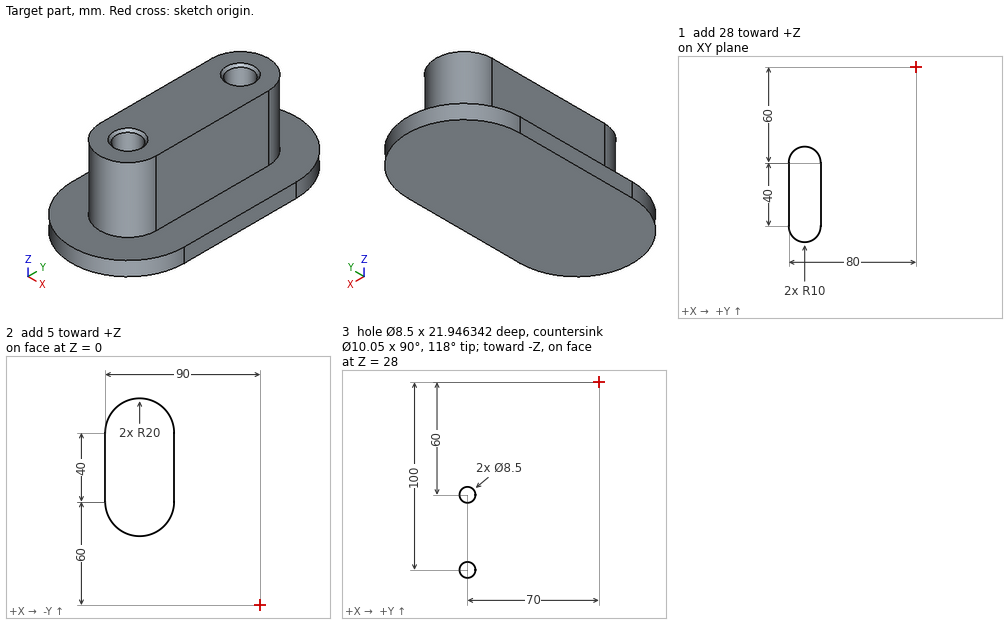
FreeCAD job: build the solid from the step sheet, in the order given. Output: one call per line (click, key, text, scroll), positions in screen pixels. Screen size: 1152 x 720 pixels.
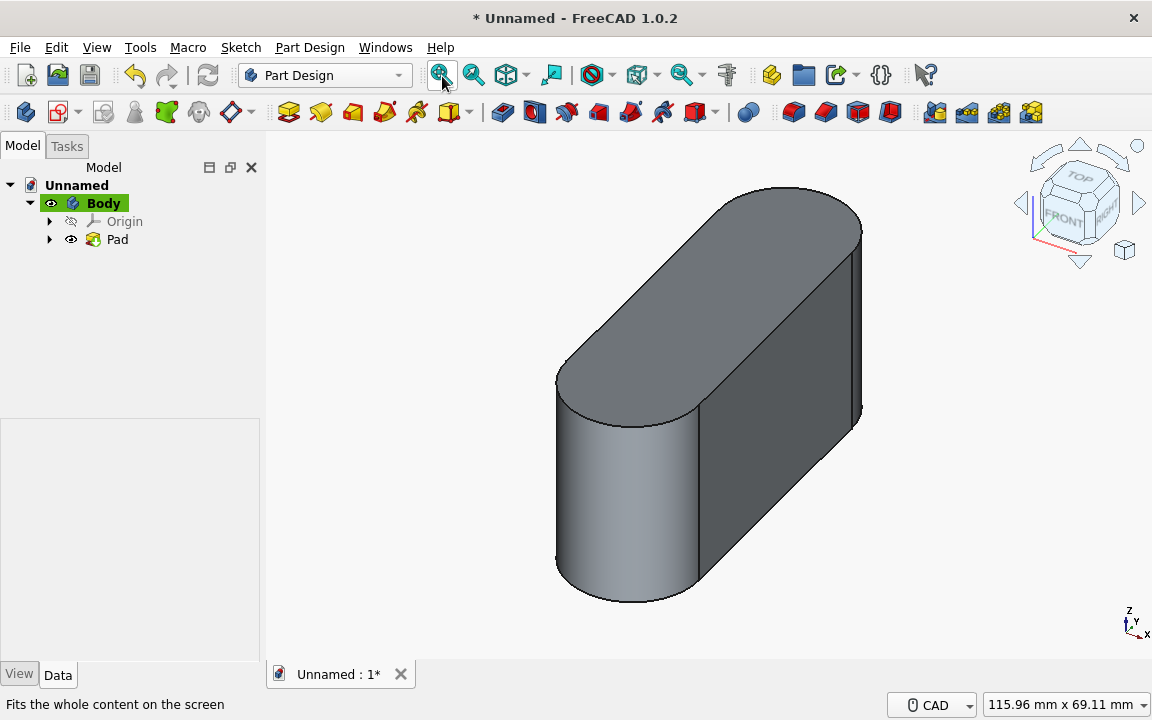
key(5)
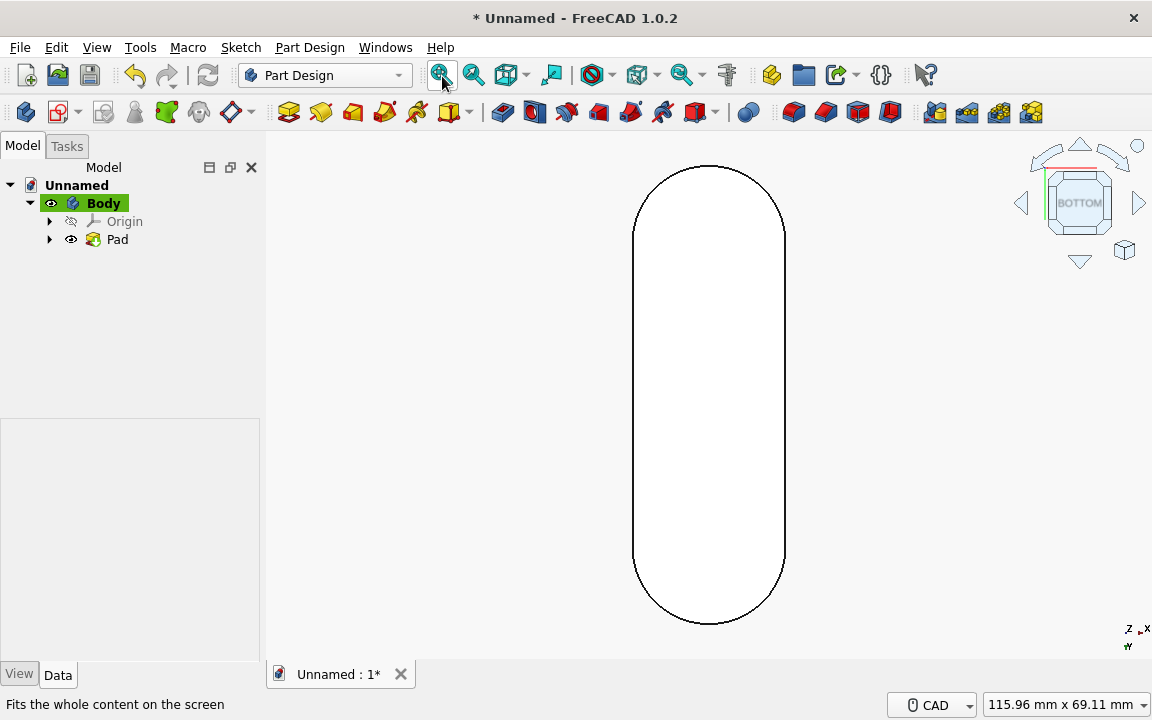
click(709, 525)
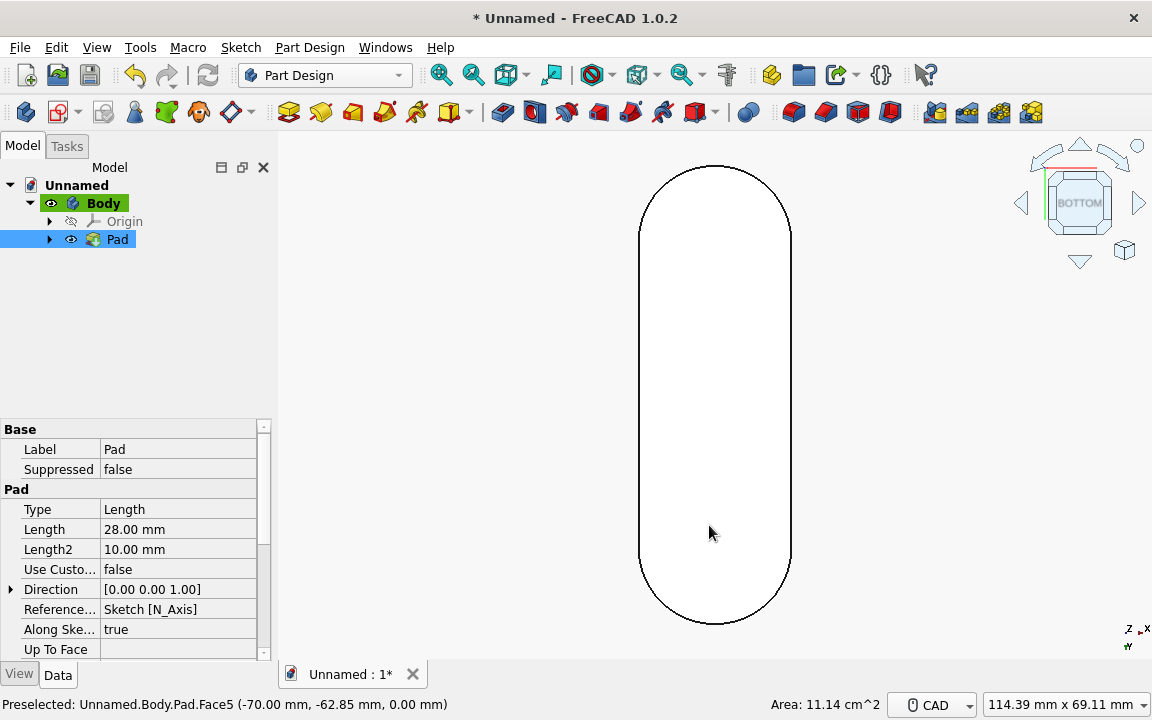
click(58, 112)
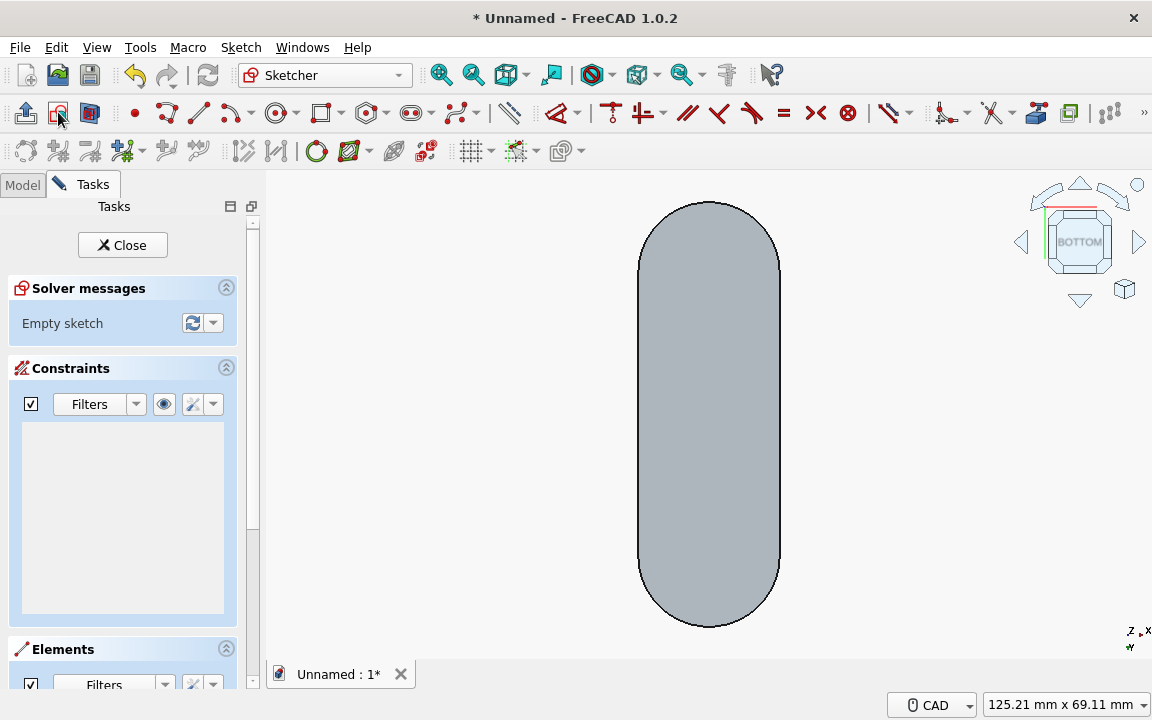
scroll(498, 332, down, 5)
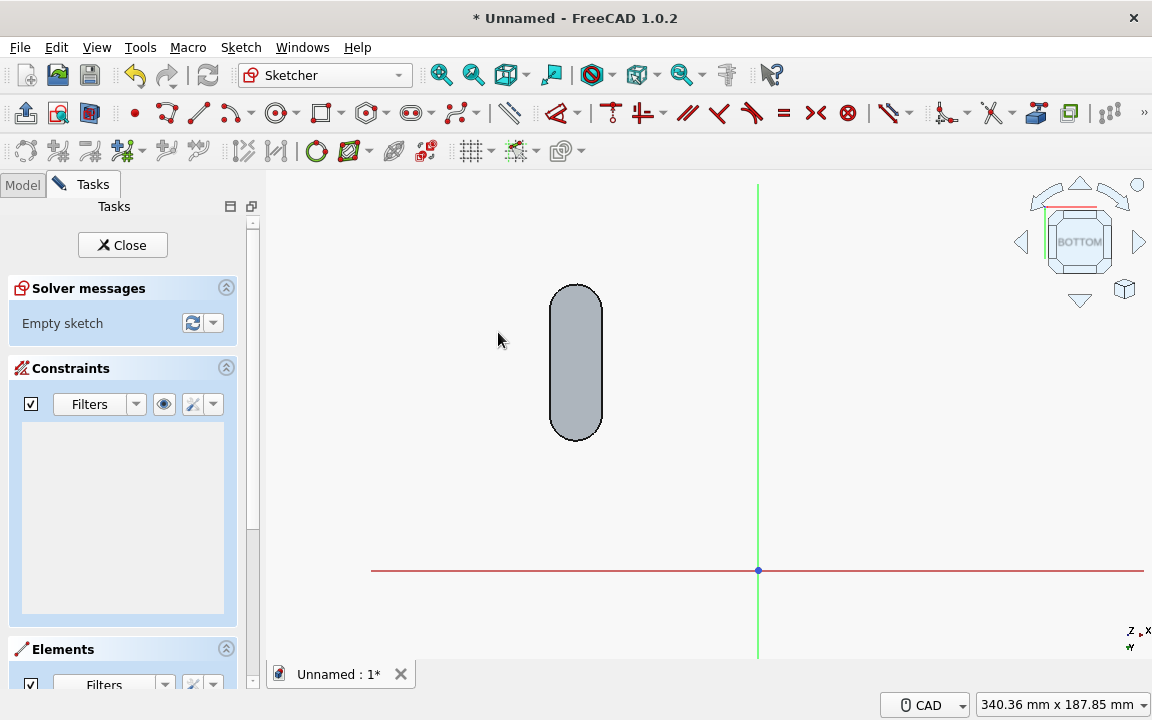
click(412, 114)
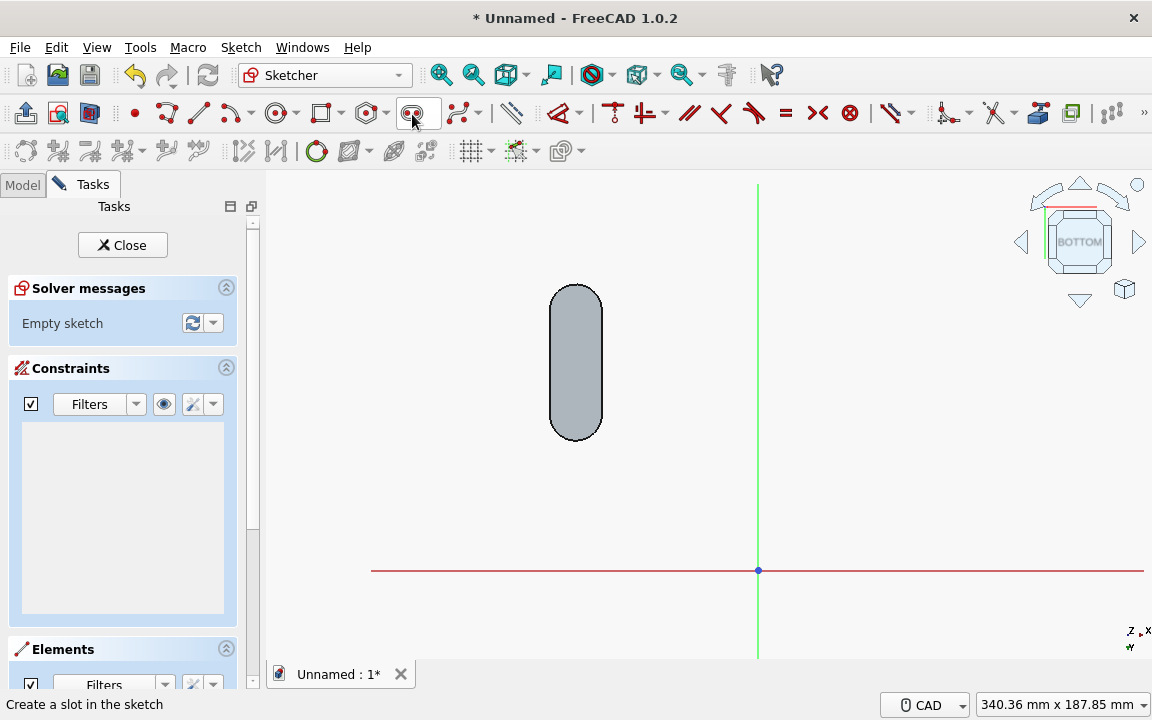
click(576, 415)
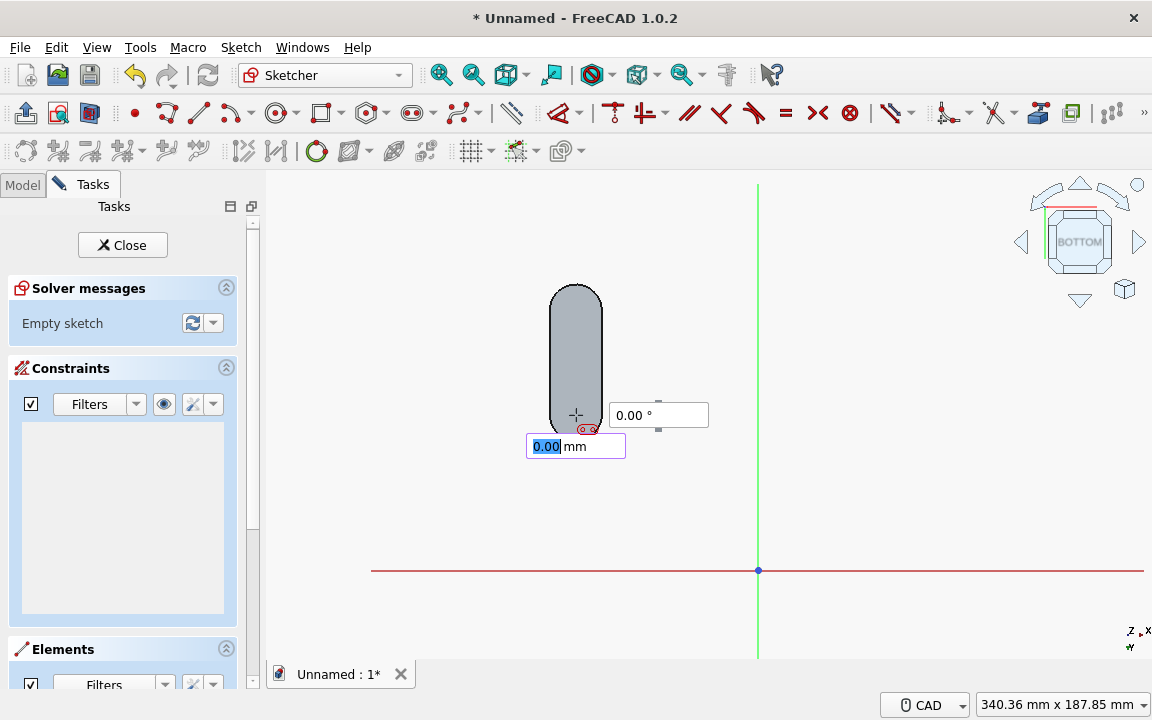
click(576, 310)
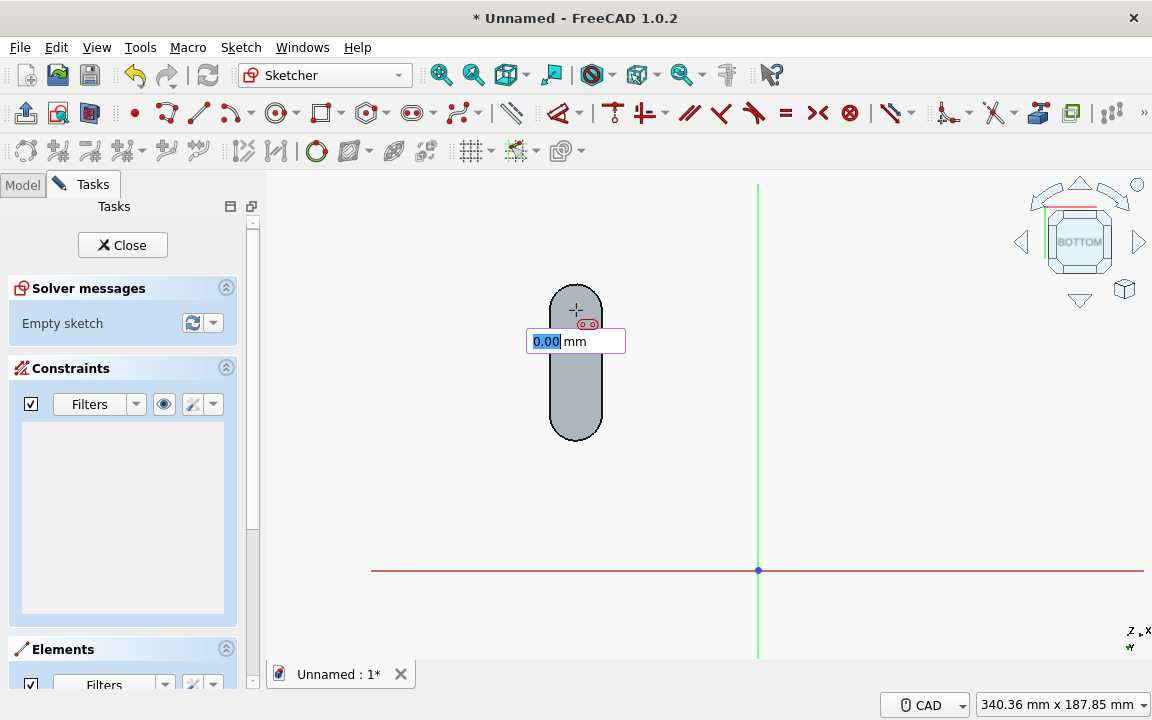
click(524, 363)
key(Escape)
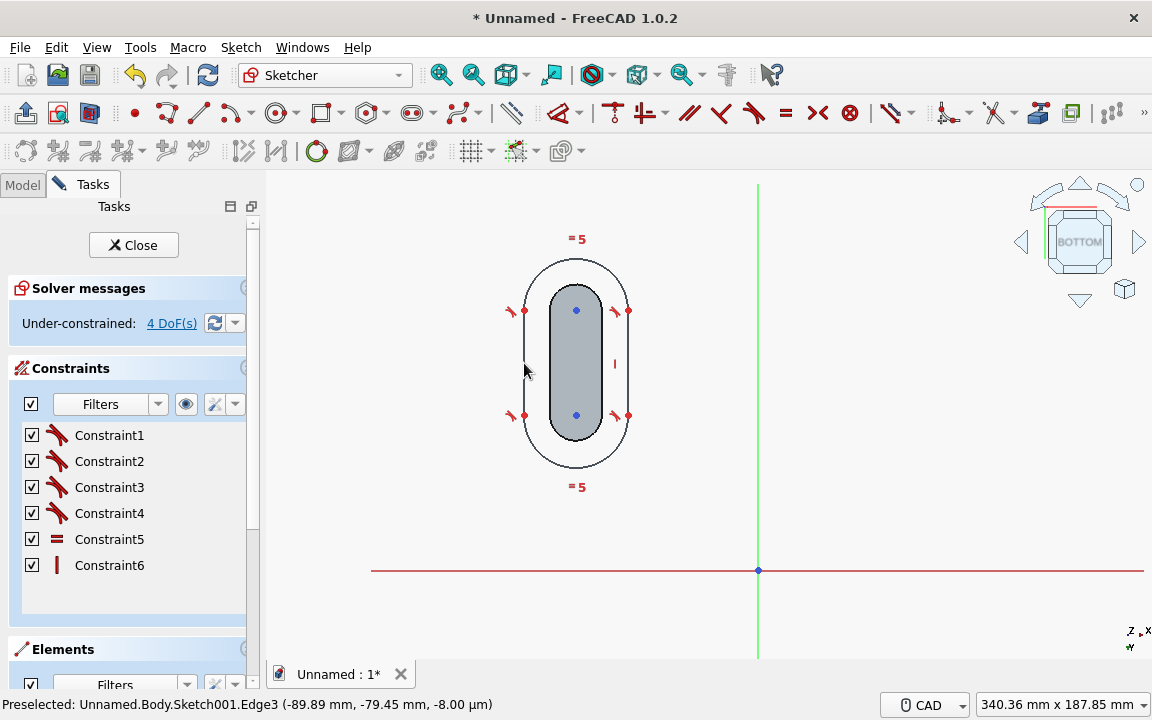
click(558, 114)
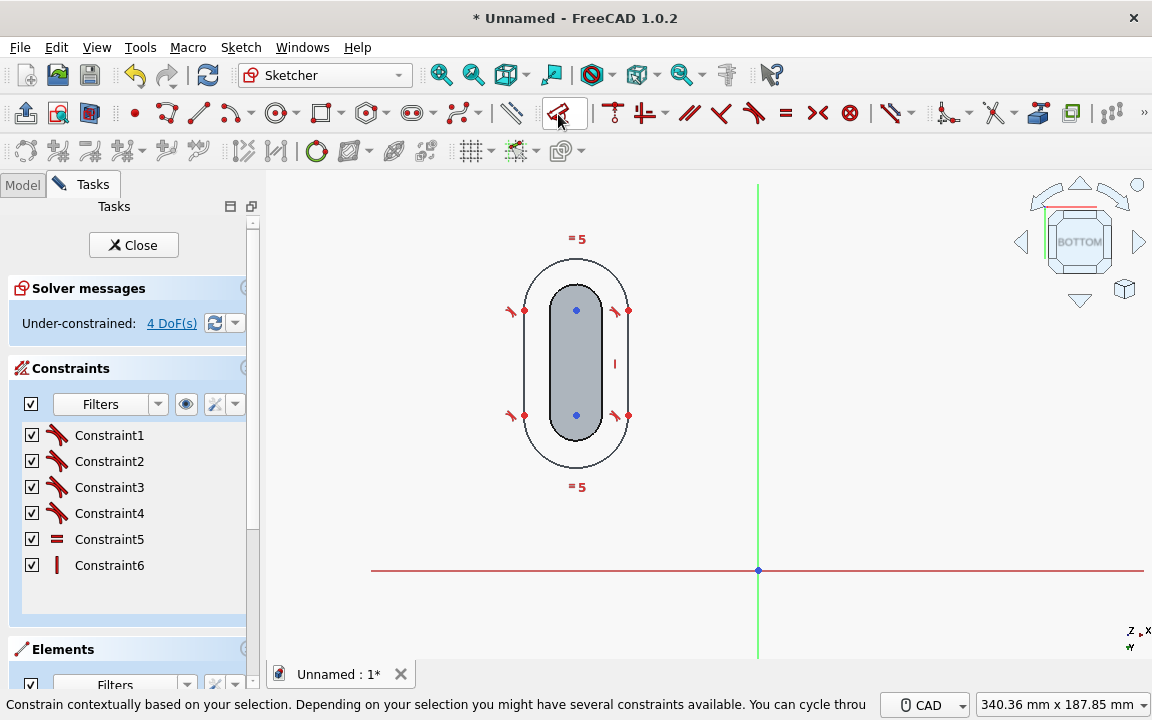
click(545, 458)
click(526, 484)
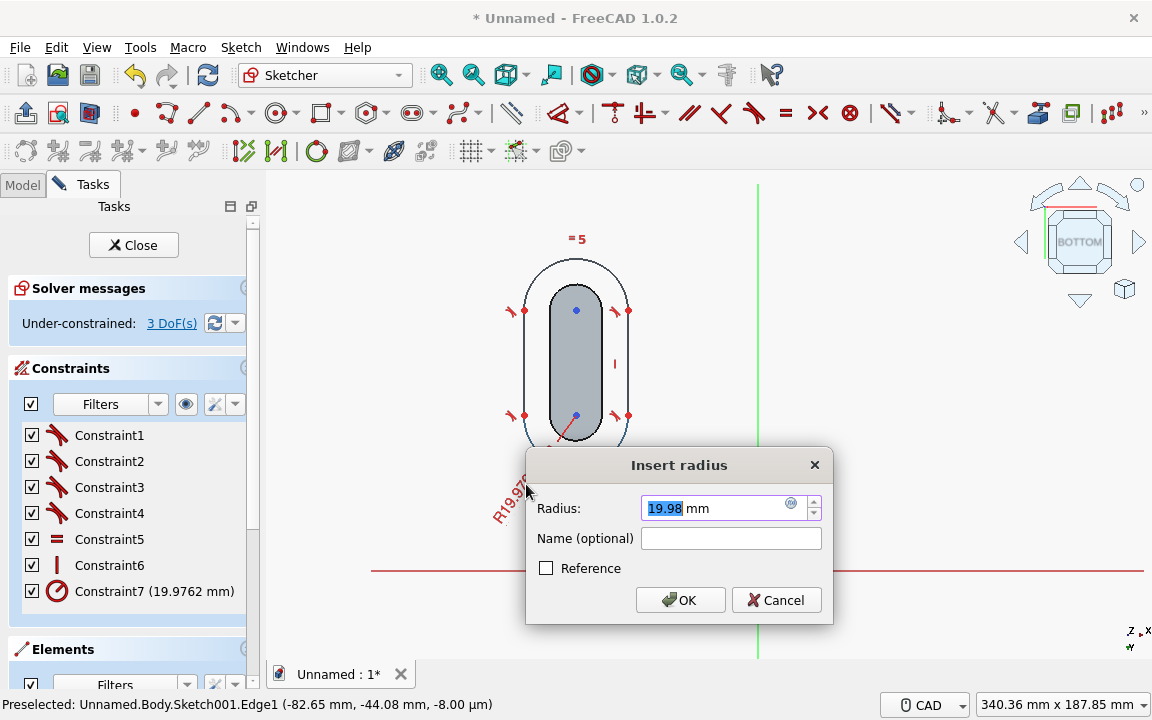
text(20)
key(Return)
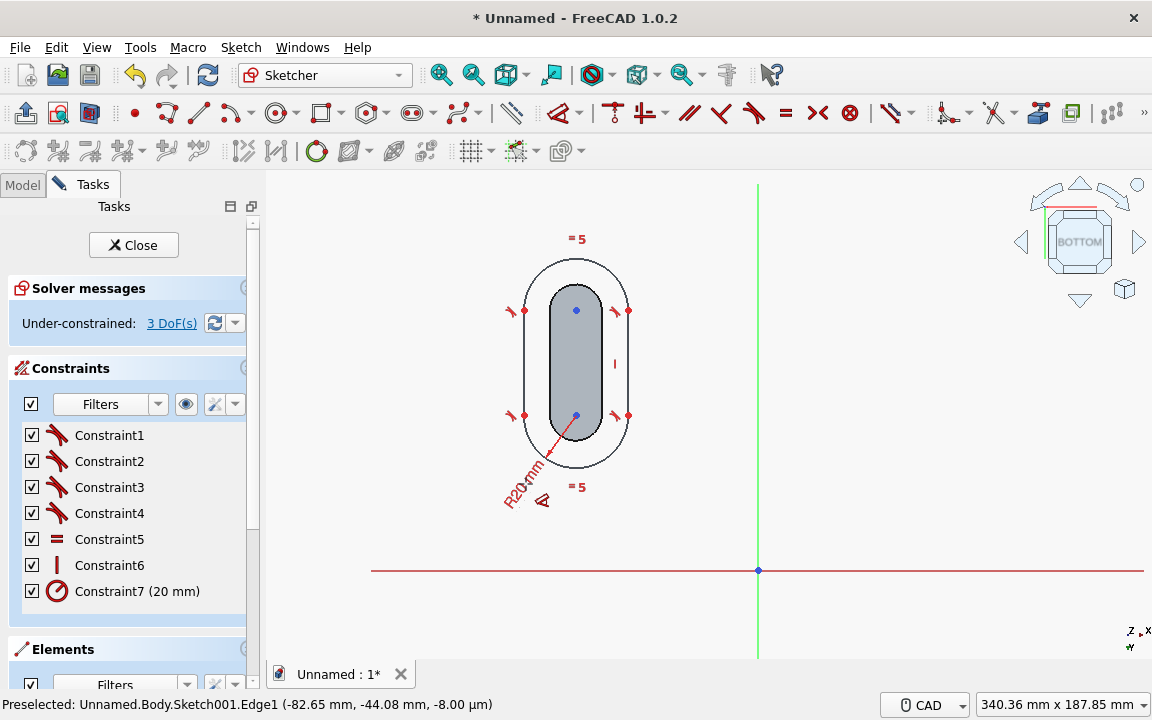
click(524, 385)
click(490, 364)